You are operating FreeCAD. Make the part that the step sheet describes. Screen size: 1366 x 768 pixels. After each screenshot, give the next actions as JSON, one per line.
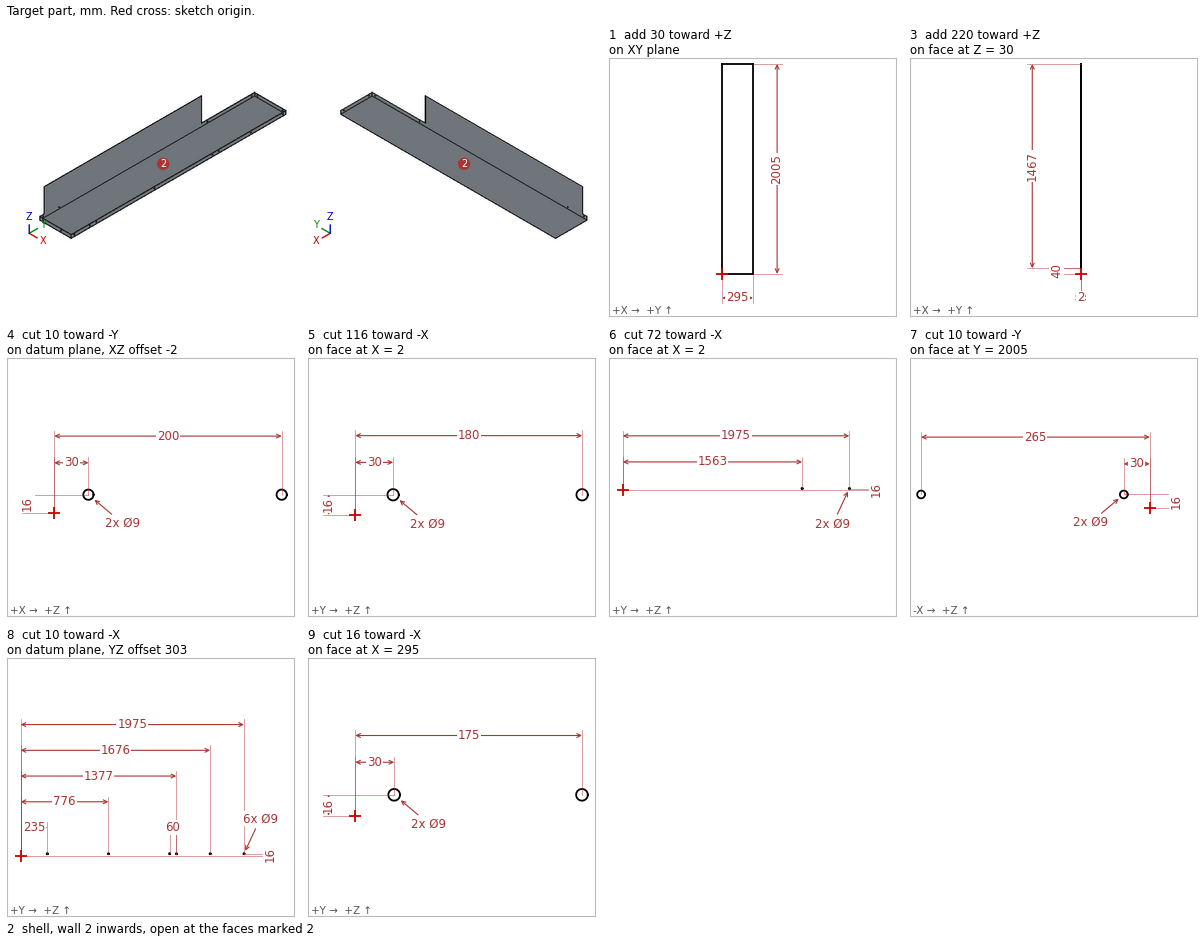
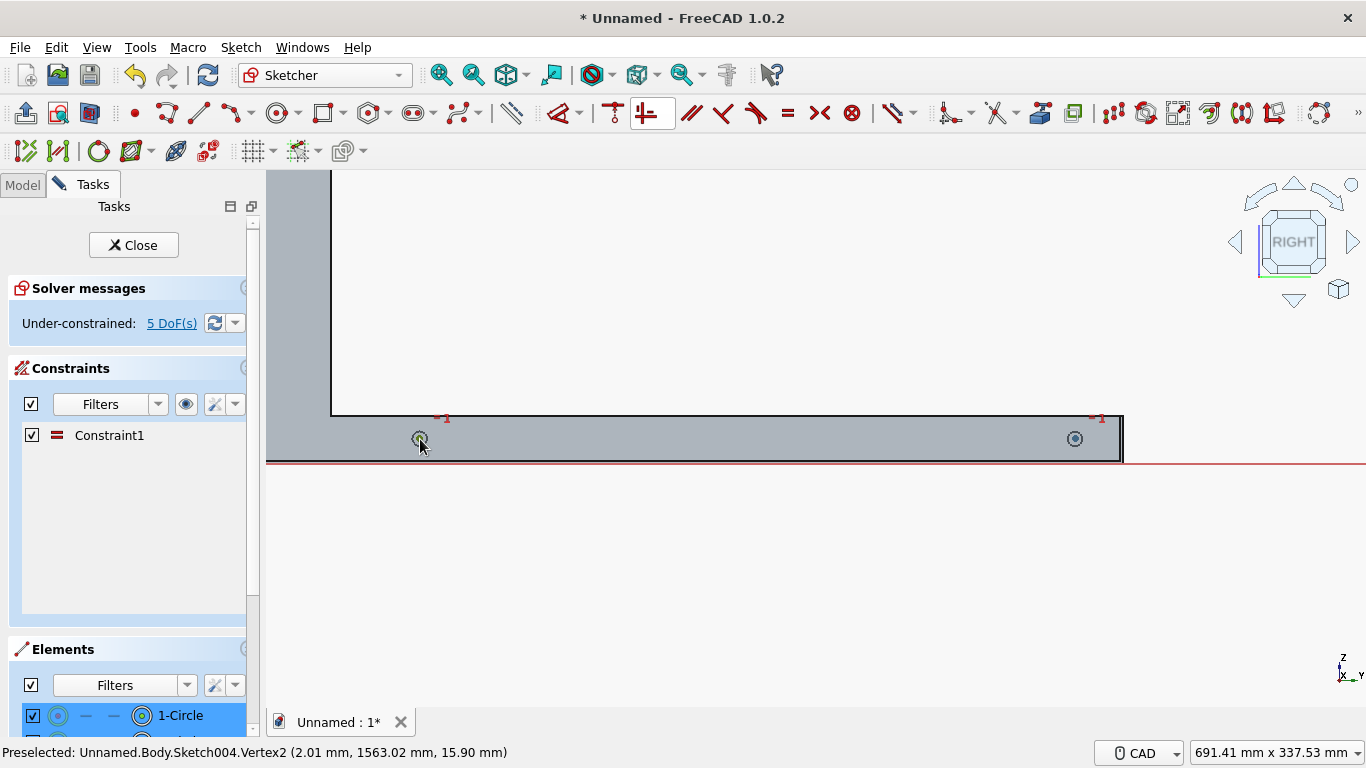
{"action": "left_click", "coordinate": [670, 114]}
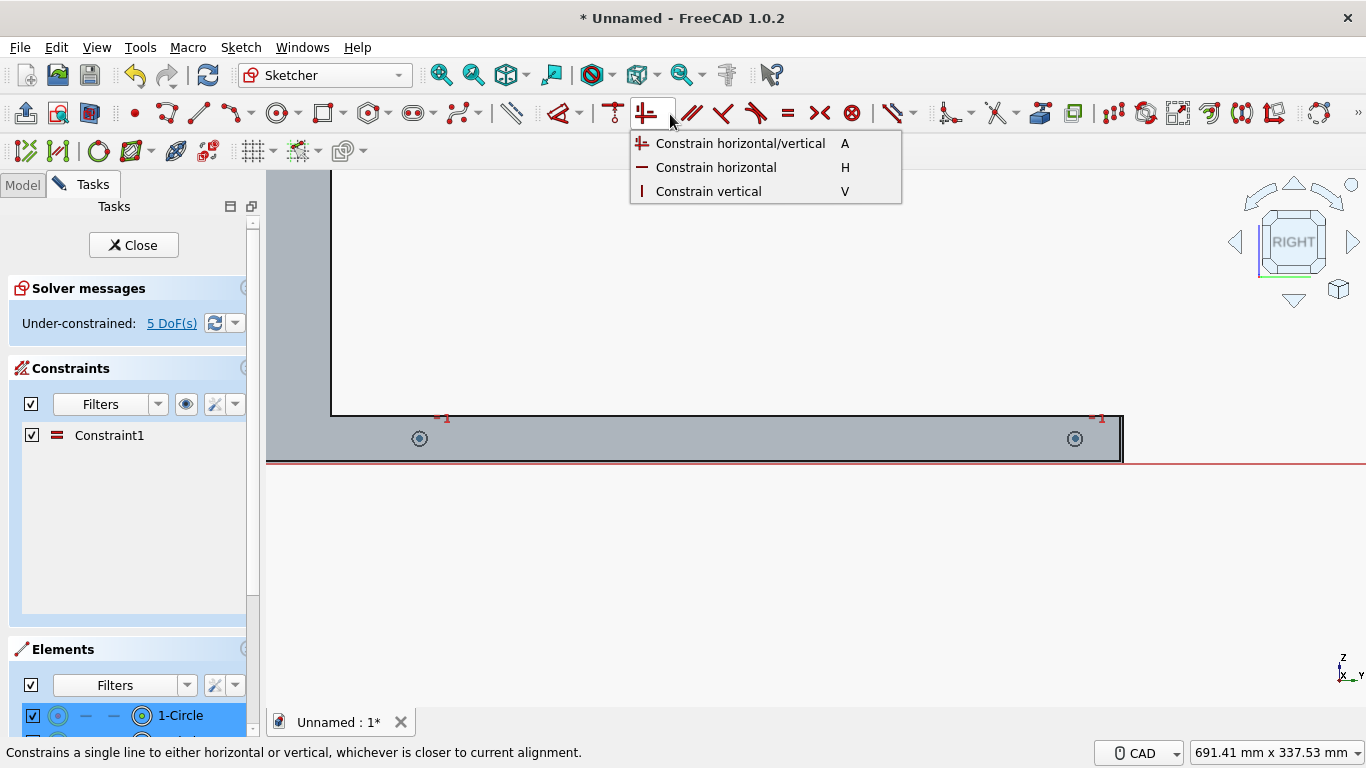
{"action": "left_click", "coordinate": [766, 167]}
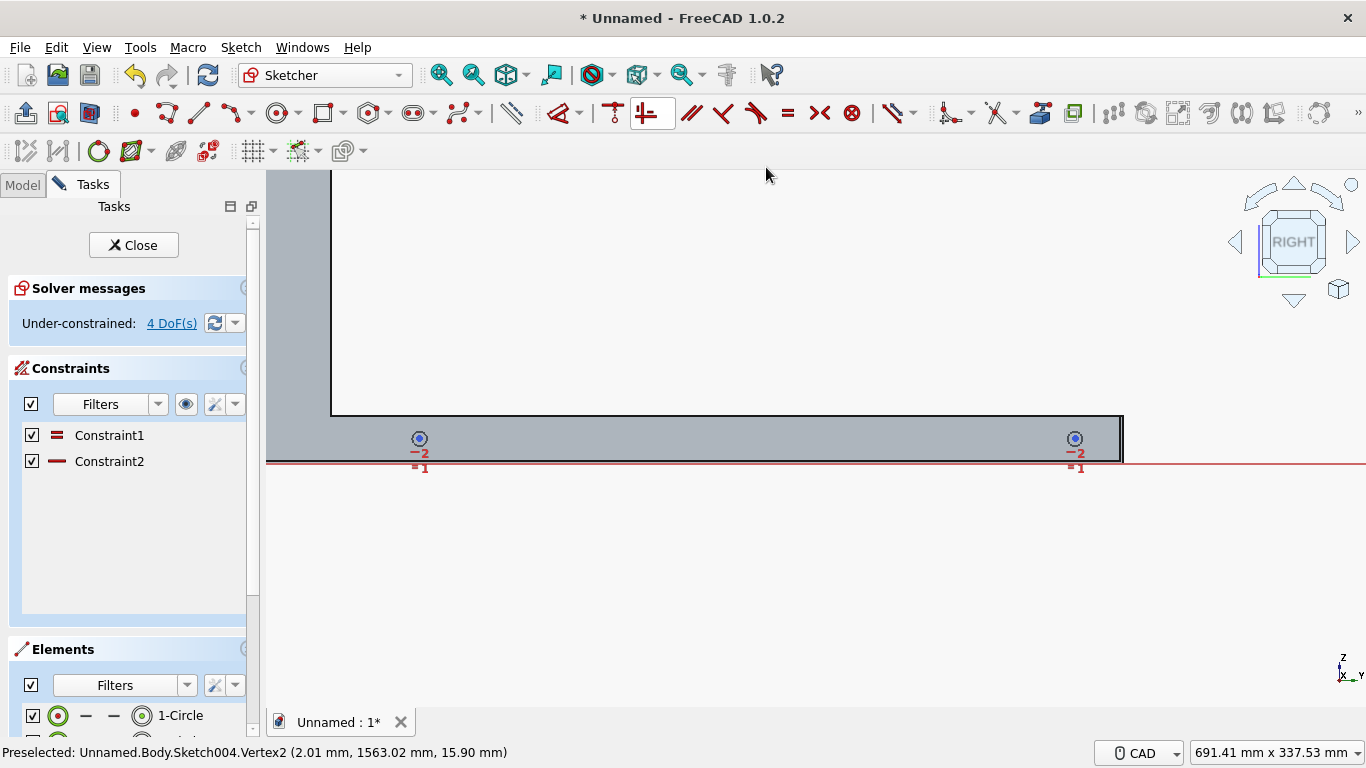
{"action": "left_click", "coordinate": [558, 114]}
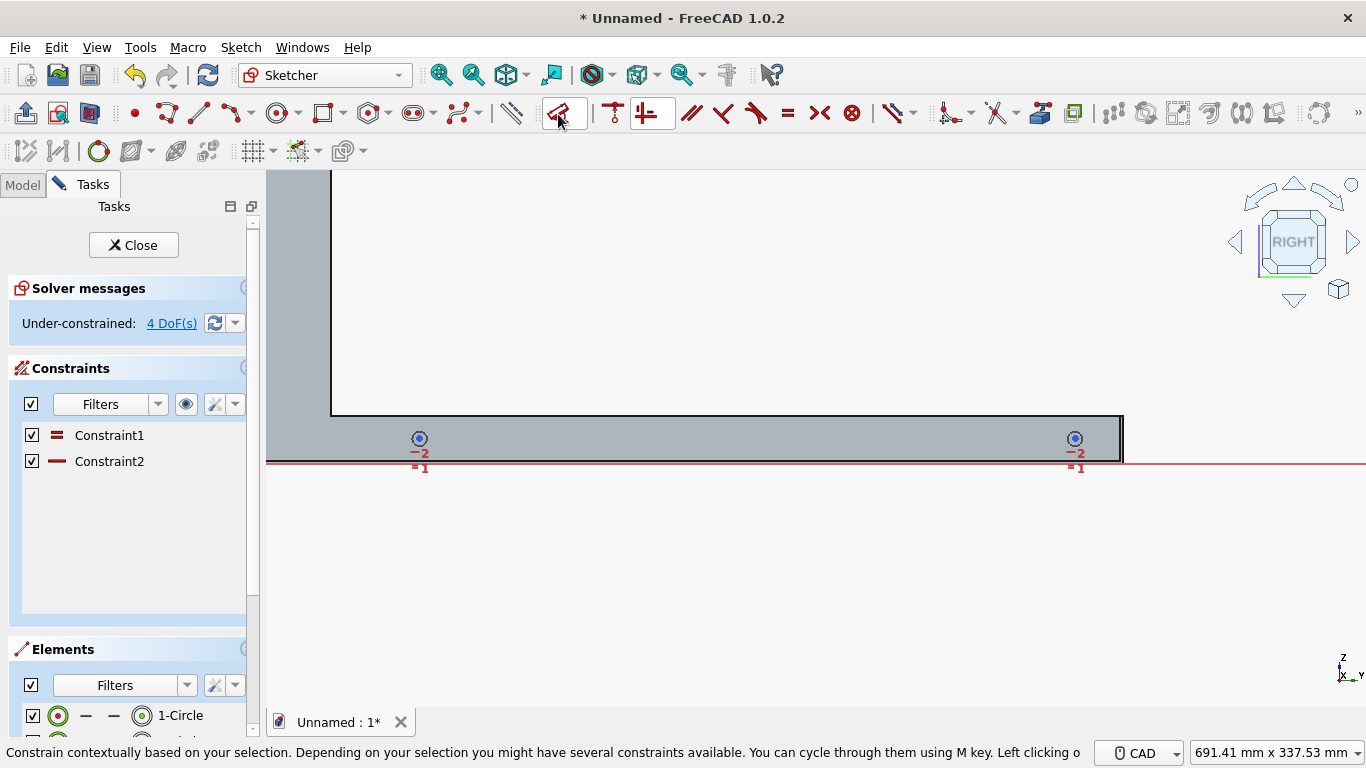
{"action": "scroll", "coordinate": [1080, 444], "scroll_direction": "up", "scroll_amount": 6}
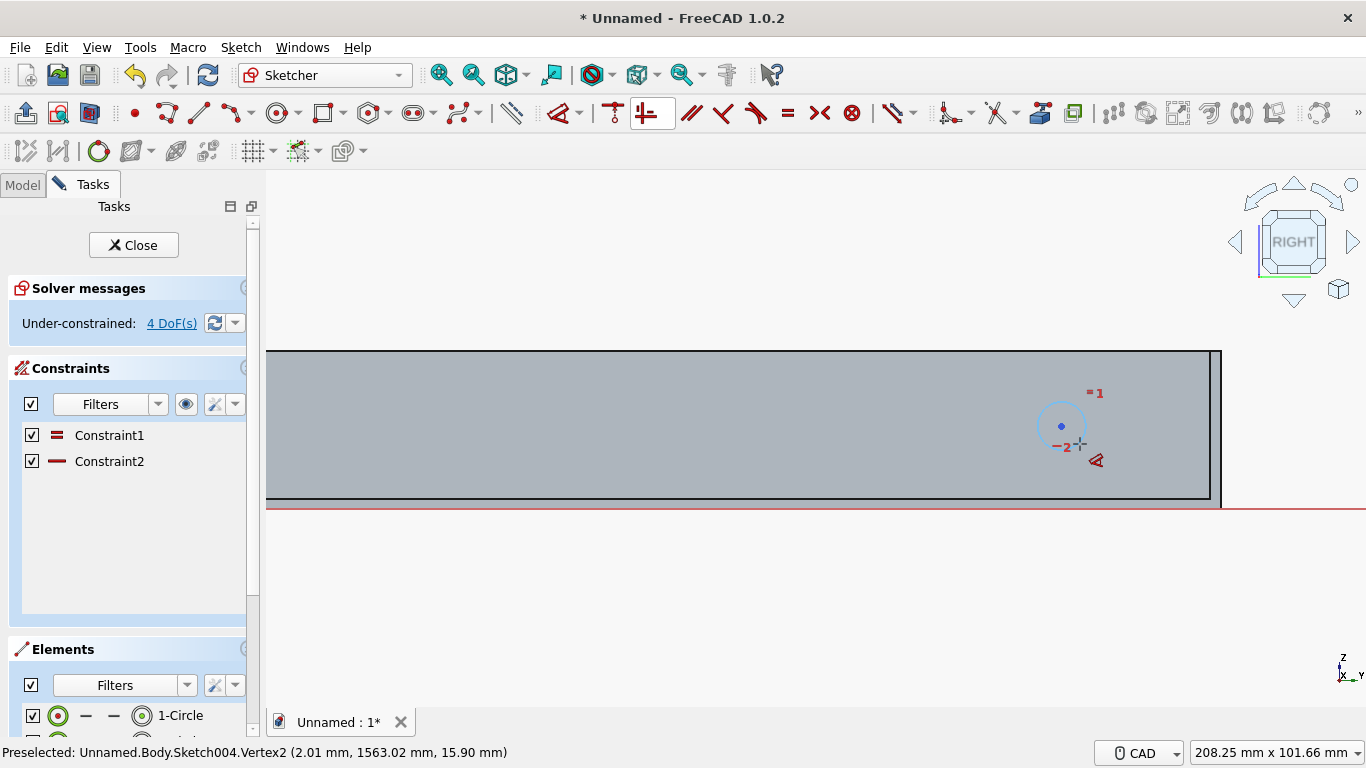
{"action": "left_click", "coordinate": [1079, 443]}
{"action": "left_click", "coordinate": [1102, 465]}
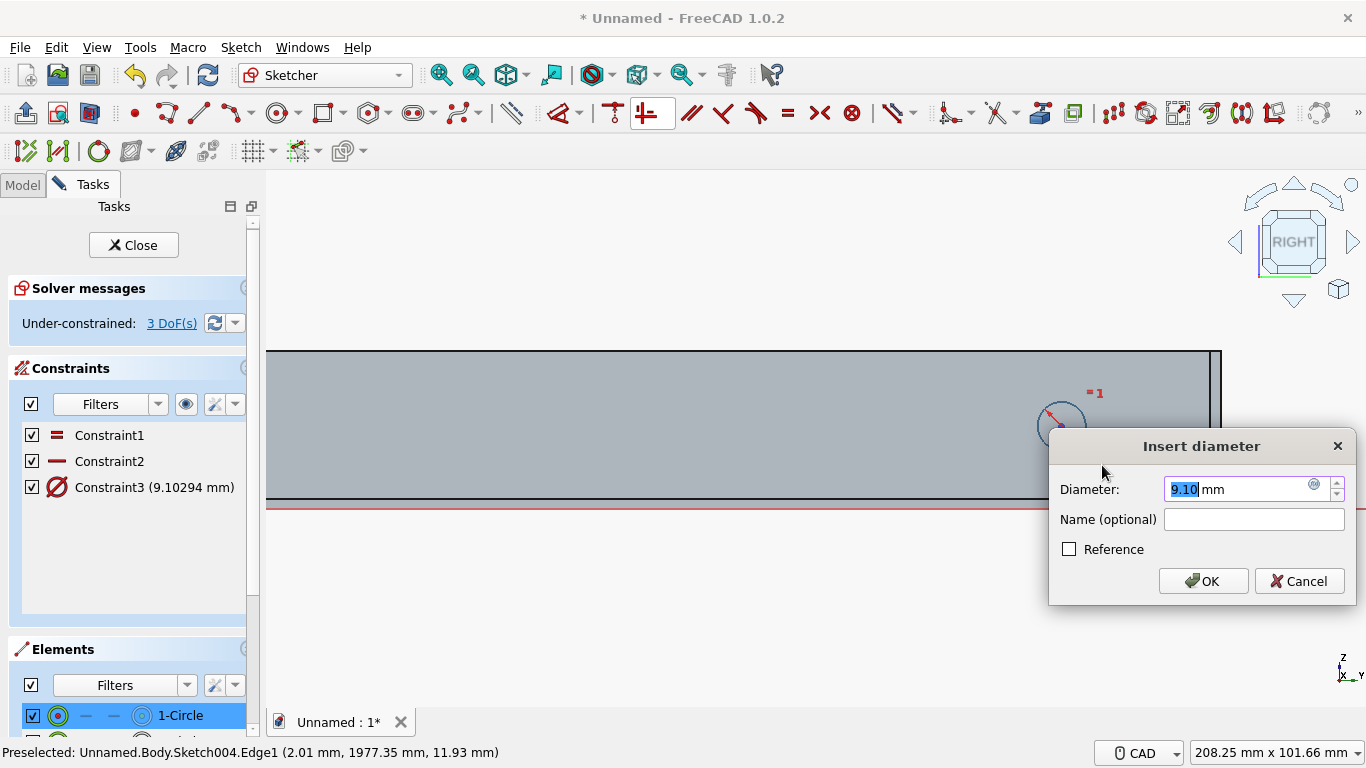
{"action": "type", "text": "9"}
{"action": "key", "text": "Return"}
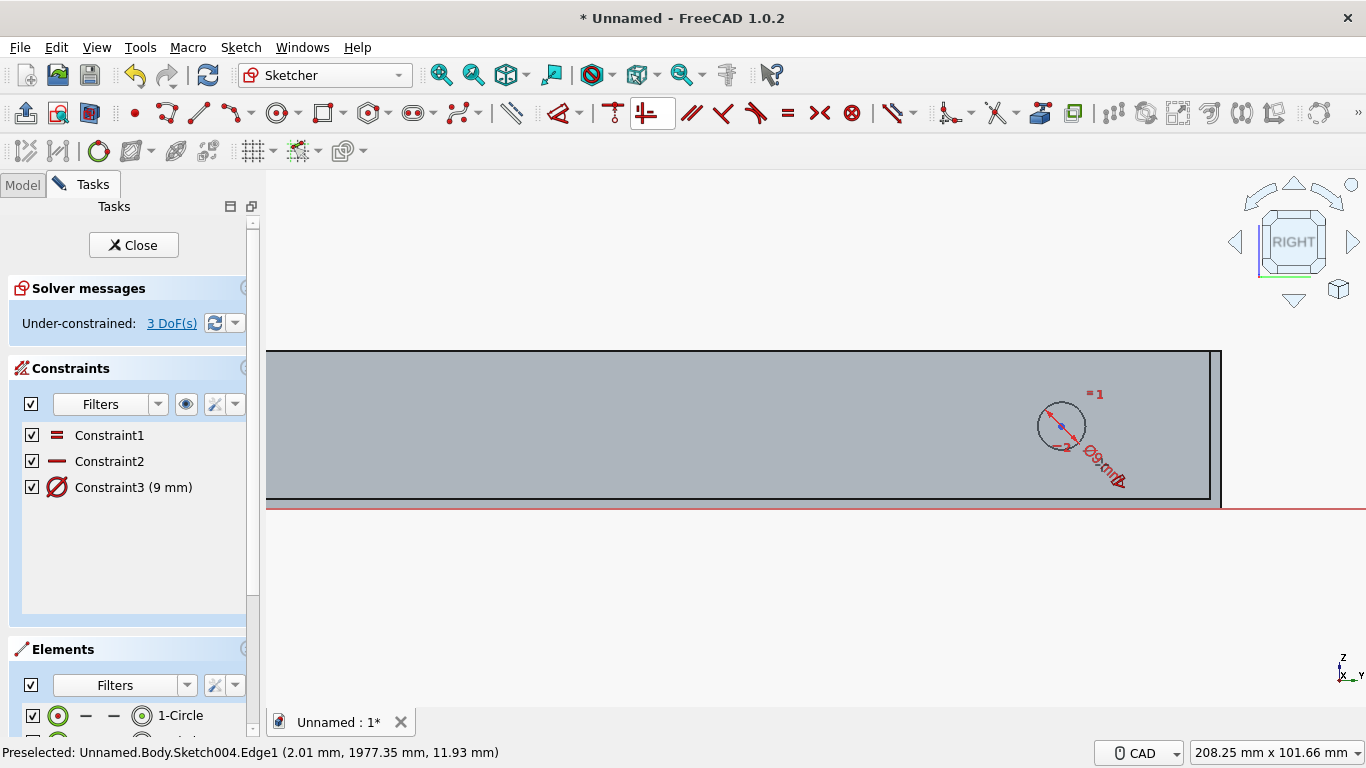
{"action": "left_click", "coordinate": [1062, 426]}
{"action": "left_click", "coordinate": [1096, 487]}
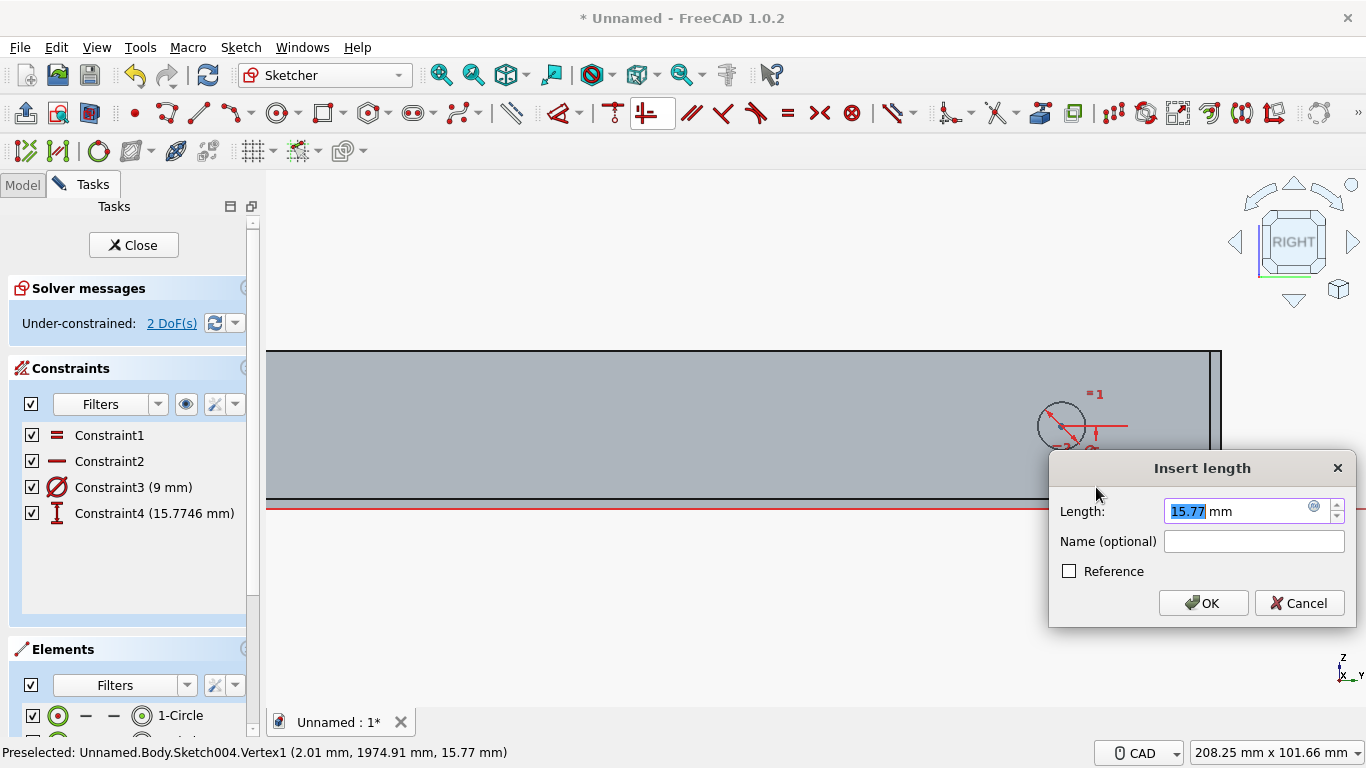
{"action": "type", "text": "16"}
{"action": "key", "text": "Return"}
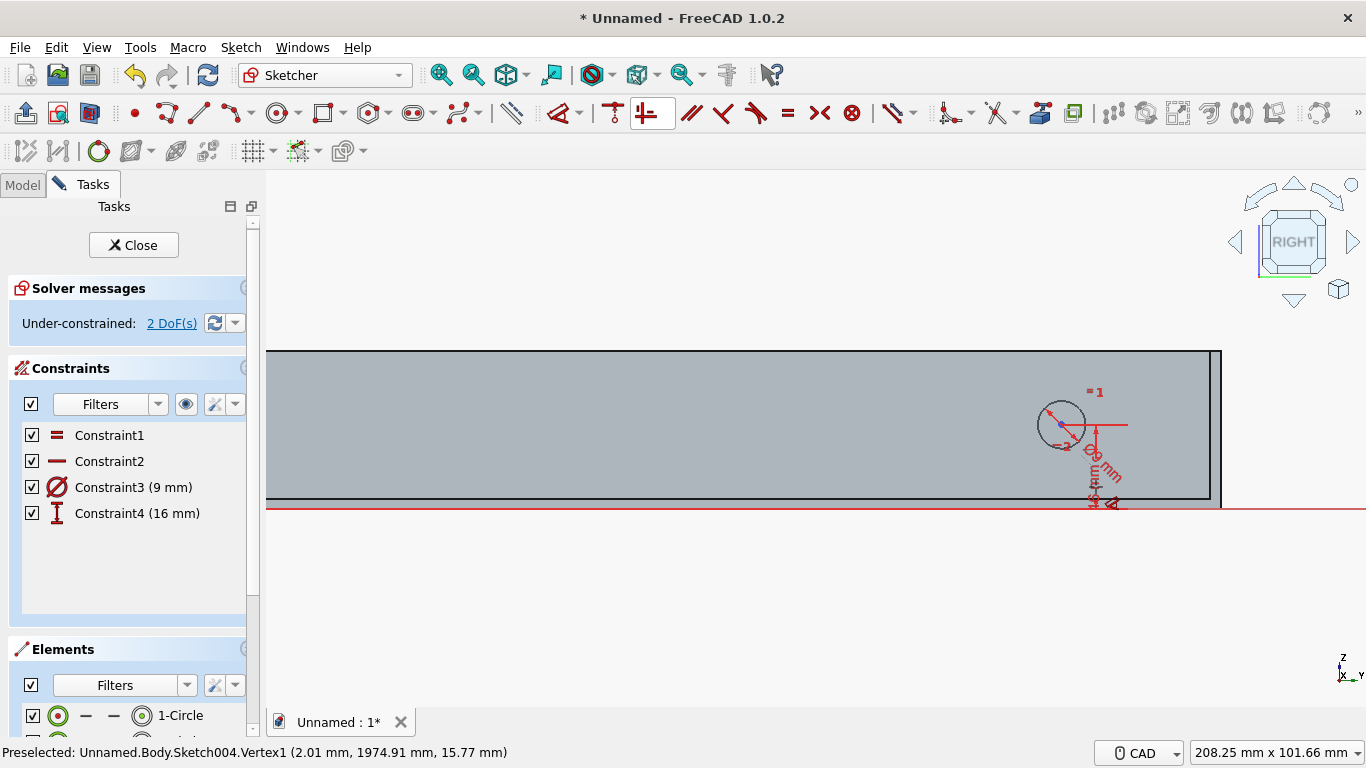
{"action": "left_click", "coordinate": [1062, 425]}
{"action": "left_click", "coordinate": [678, 543]}